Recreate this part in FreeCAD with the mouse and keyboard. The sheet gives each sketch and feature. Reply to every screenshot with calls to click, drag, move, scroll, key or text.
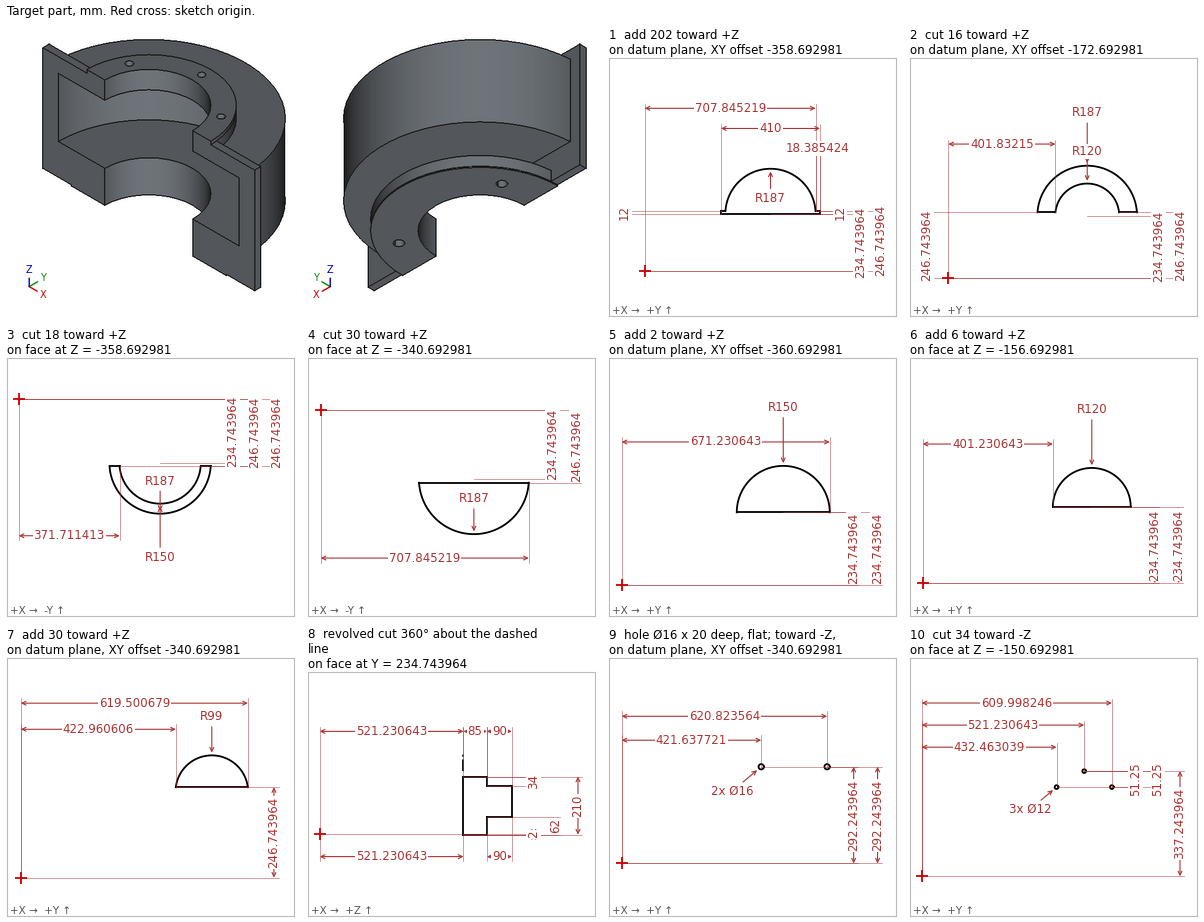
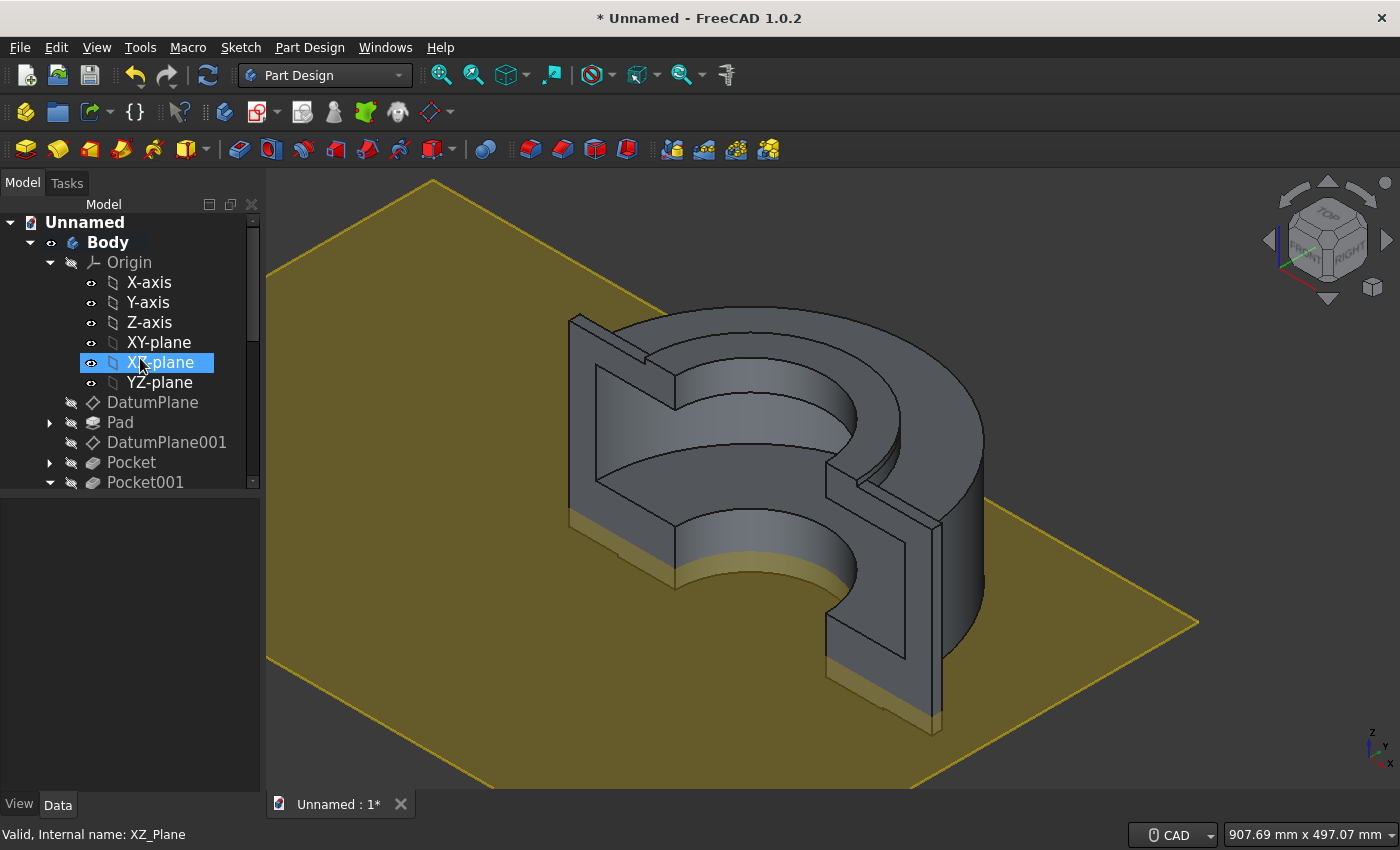
scroll(100, 358, down, 6)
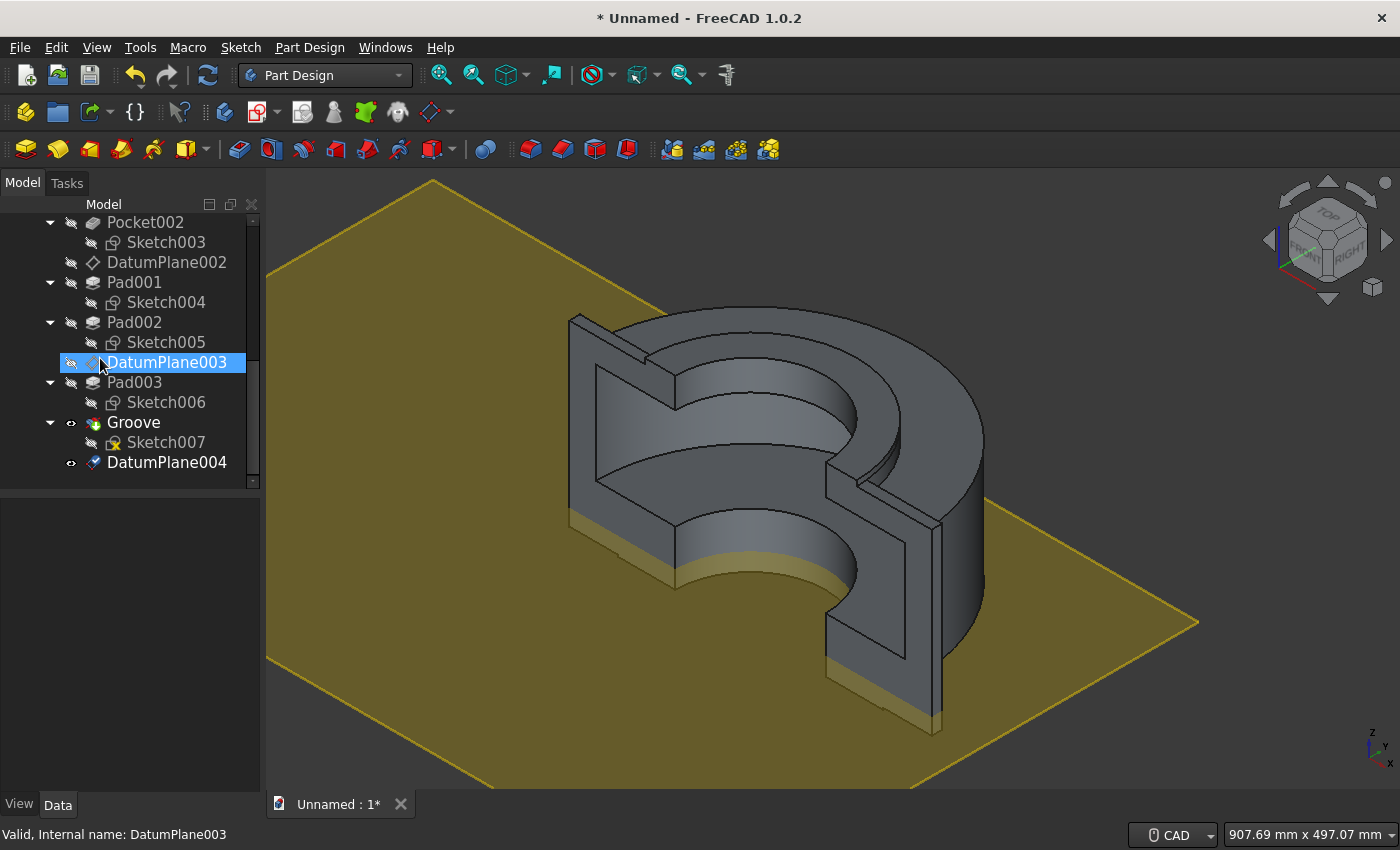
click(116, 463)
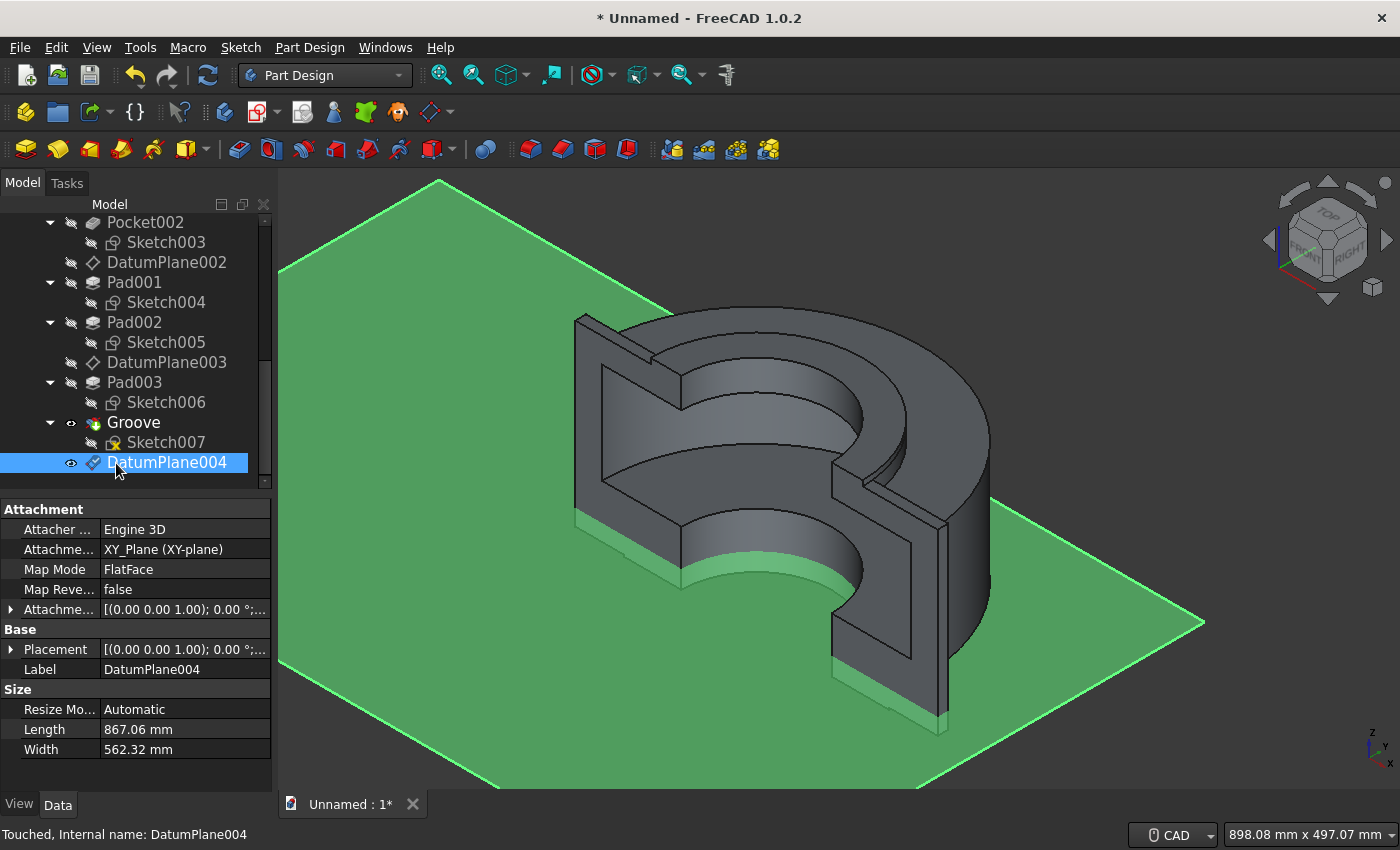
click(258, 112)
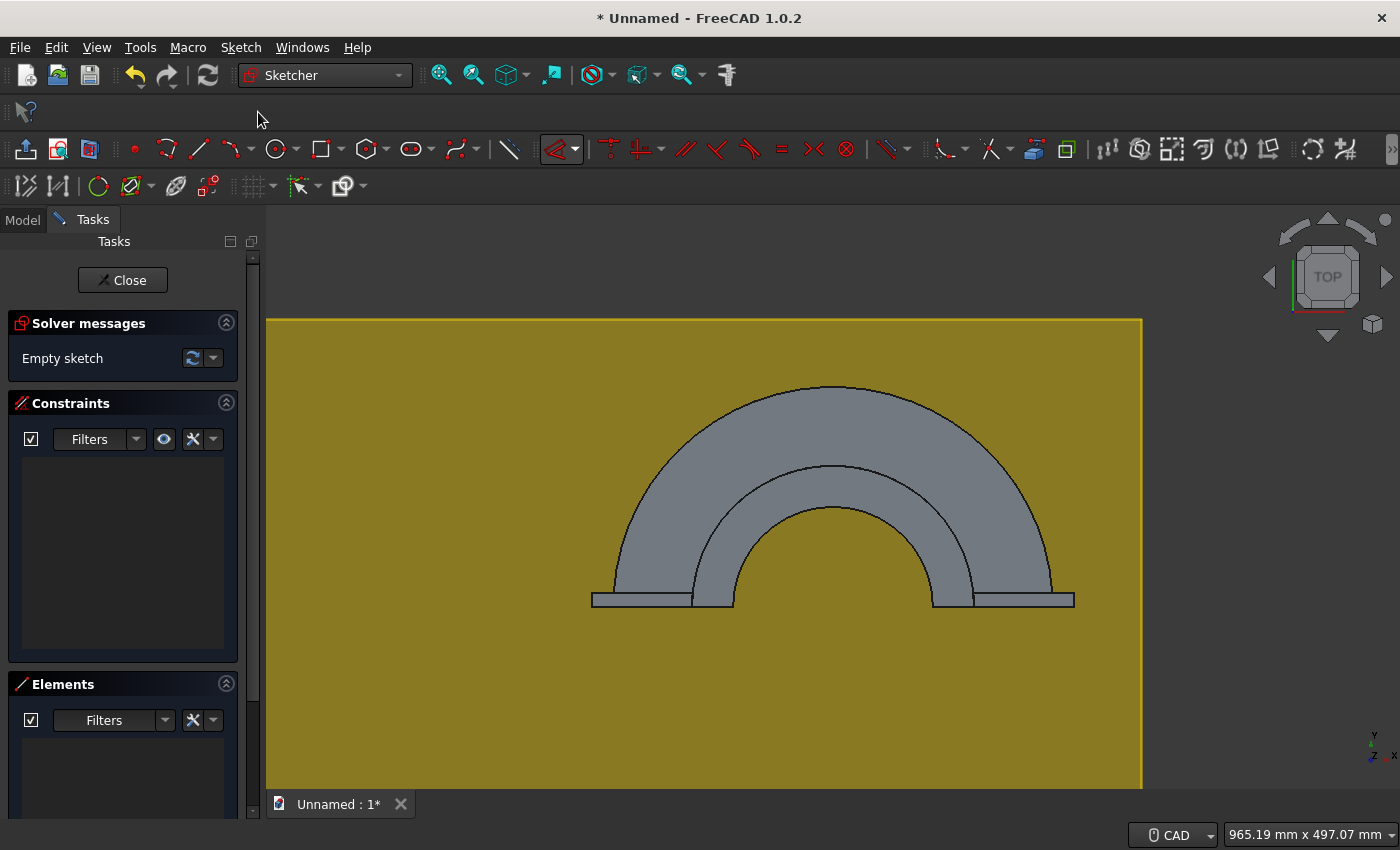
key(q)
key(s)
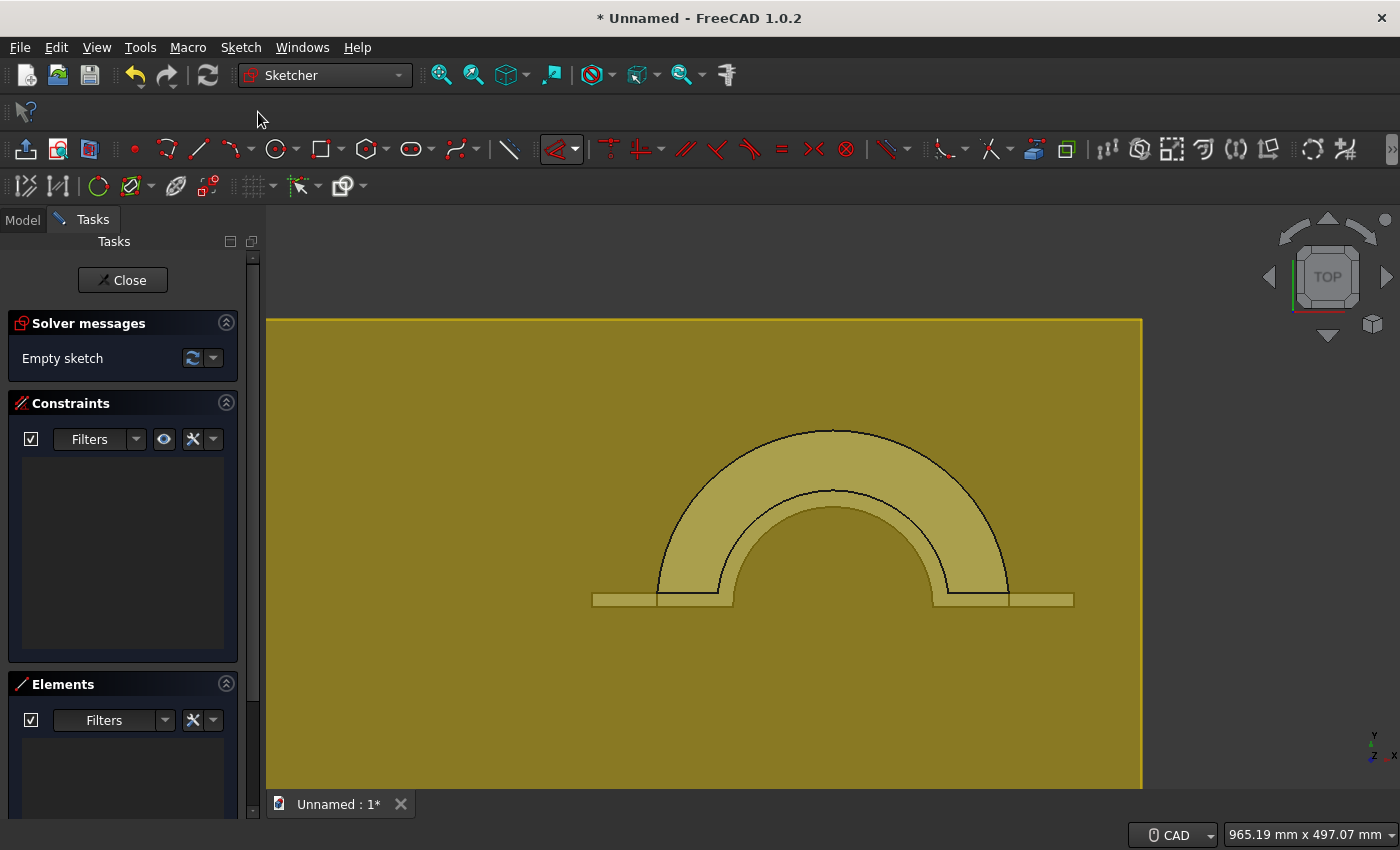
scroll(873, 564, up, 5)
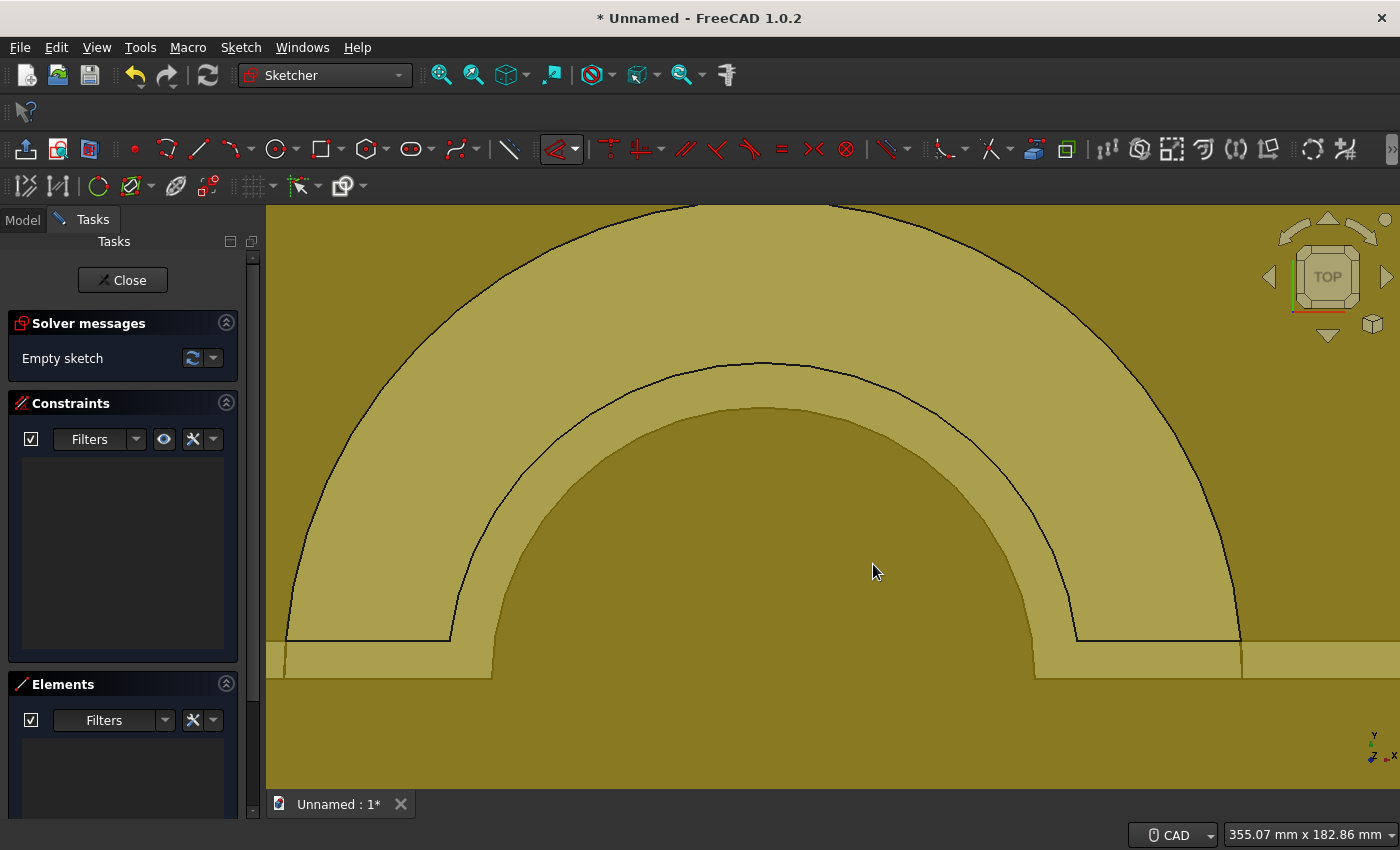
key(g)
key(c)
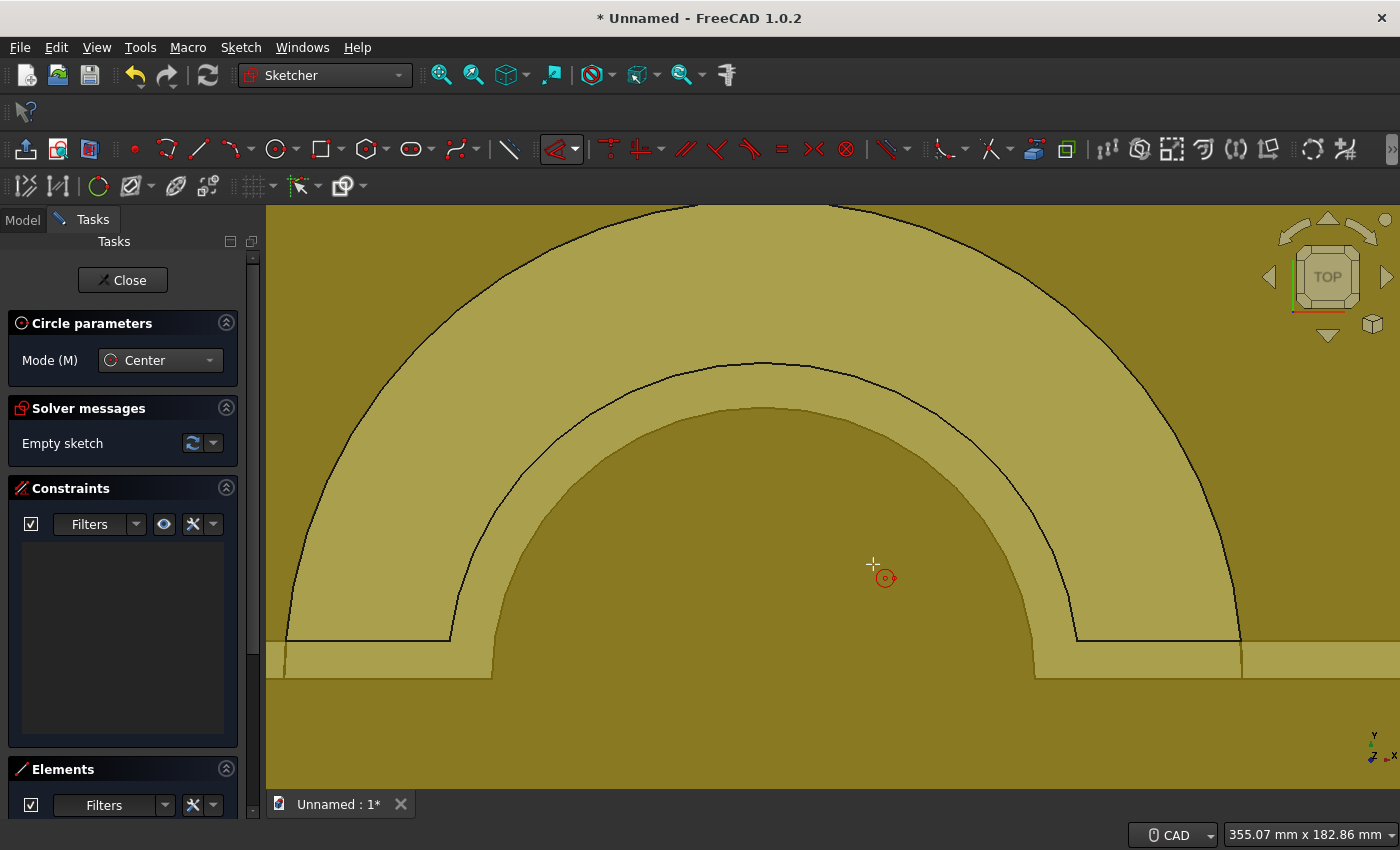
click(445, 495)
move(463, 477)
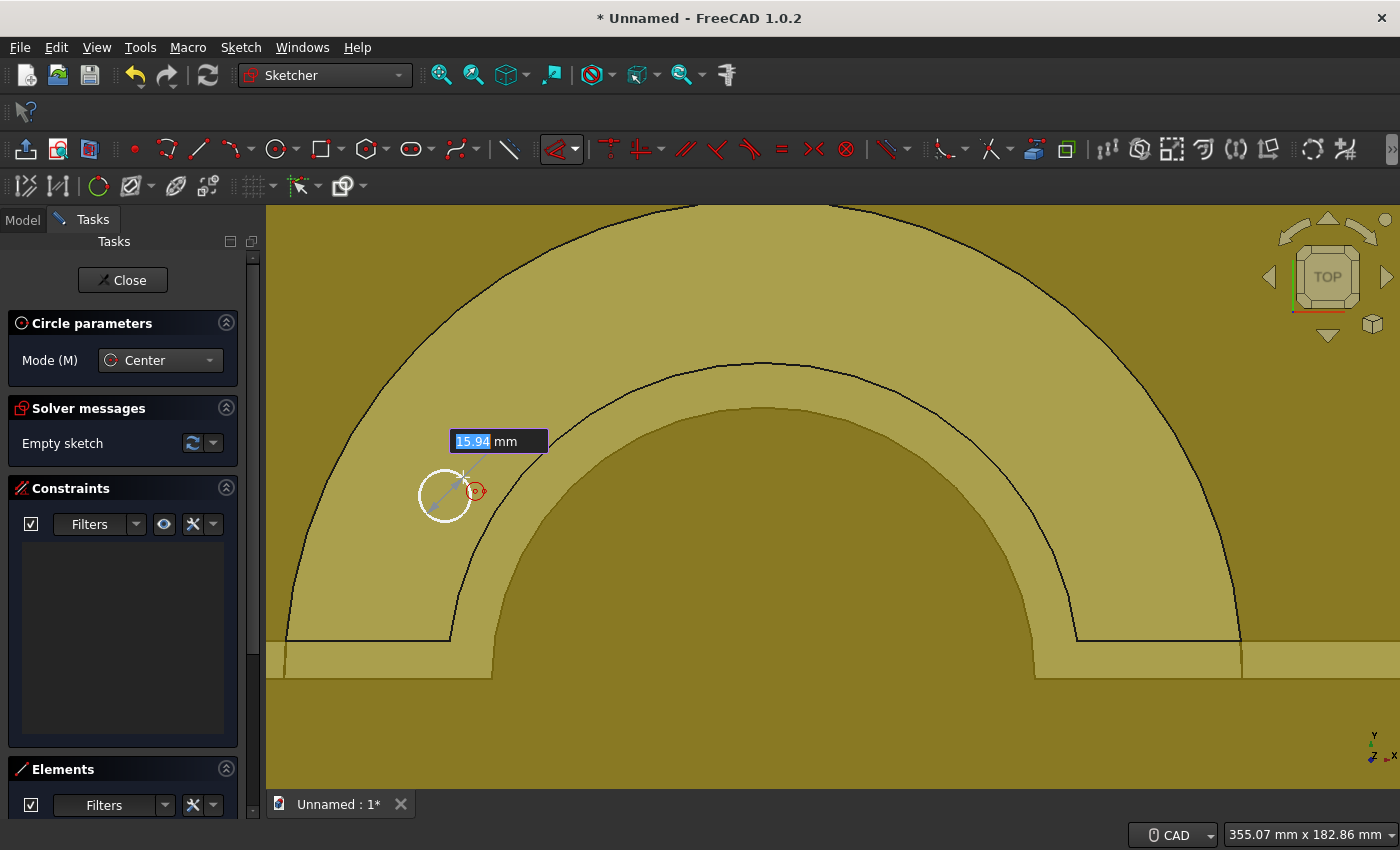
text(16)
key(Return)